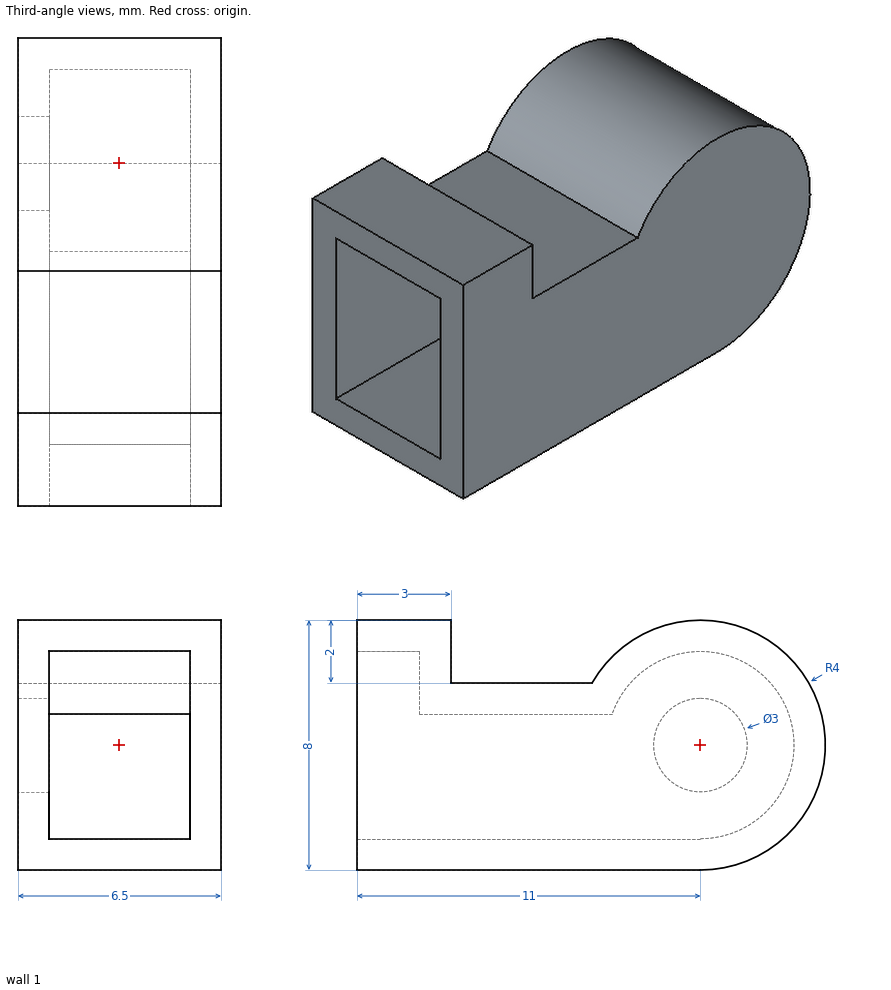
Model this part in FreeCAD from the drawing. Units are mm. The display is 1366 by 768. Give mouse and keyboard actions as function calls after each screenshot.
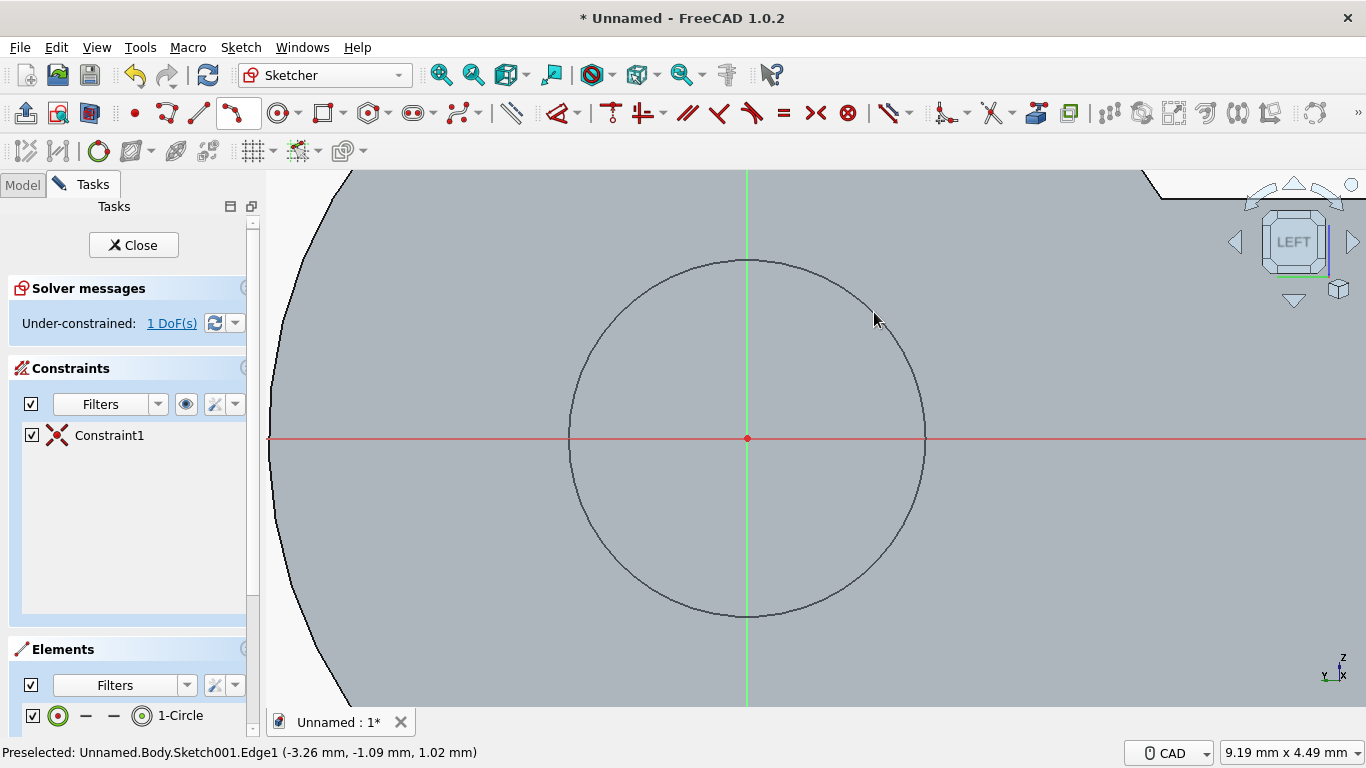
click(873, 312)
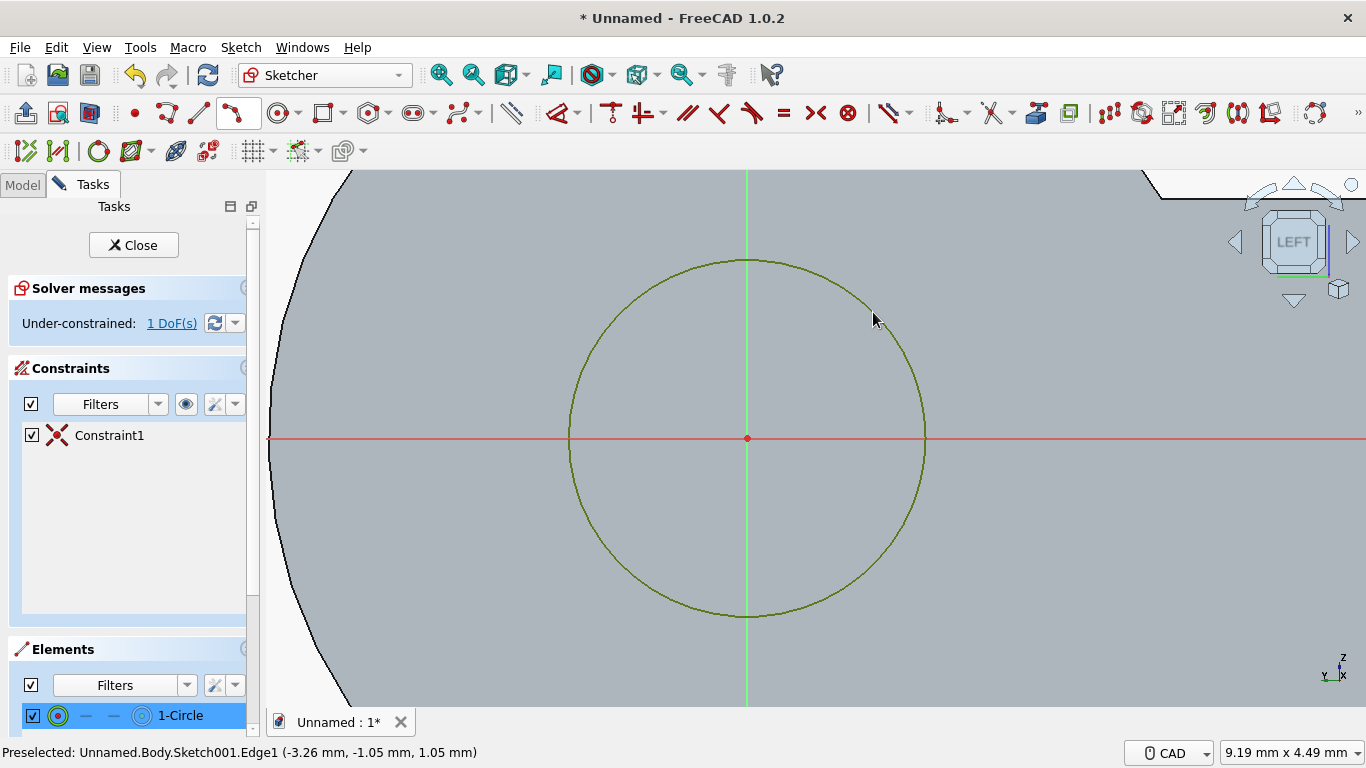
key(k)
key(o)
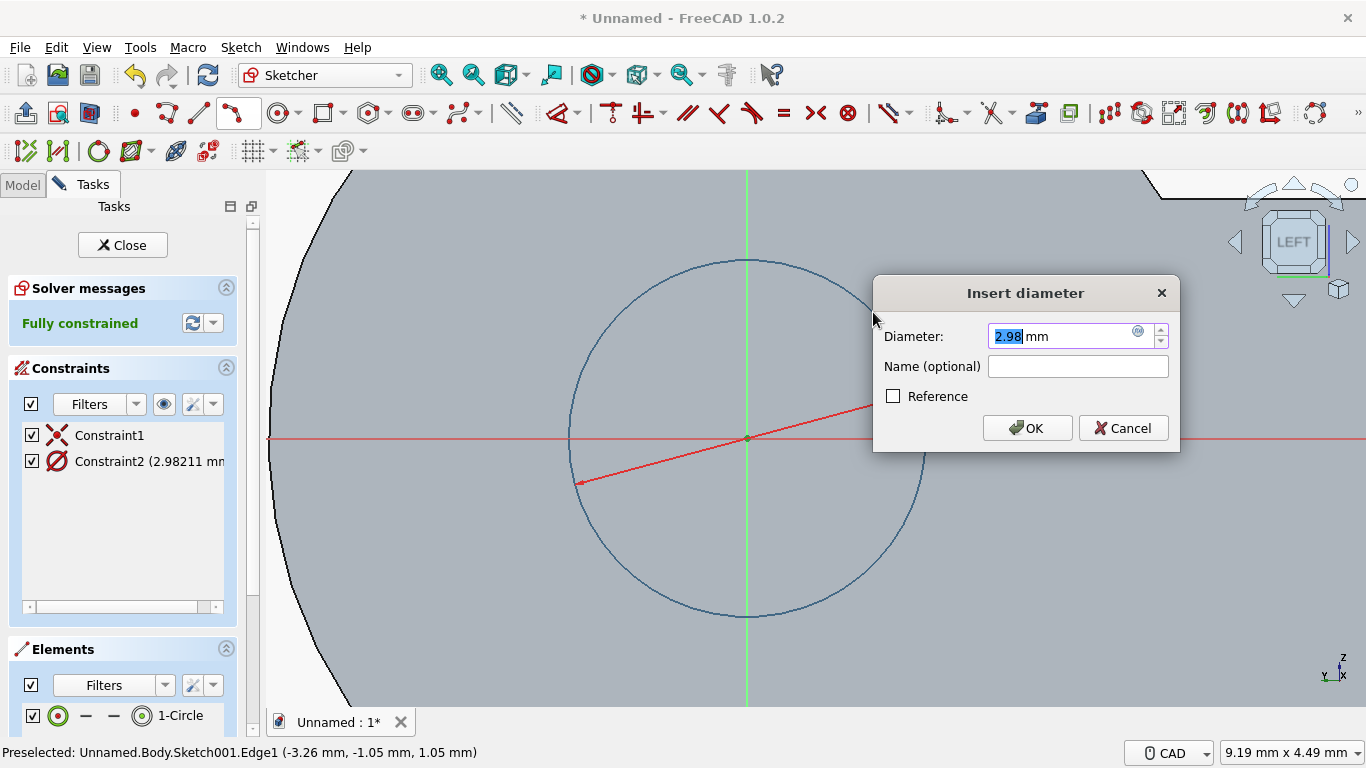
text(3)
key(Return)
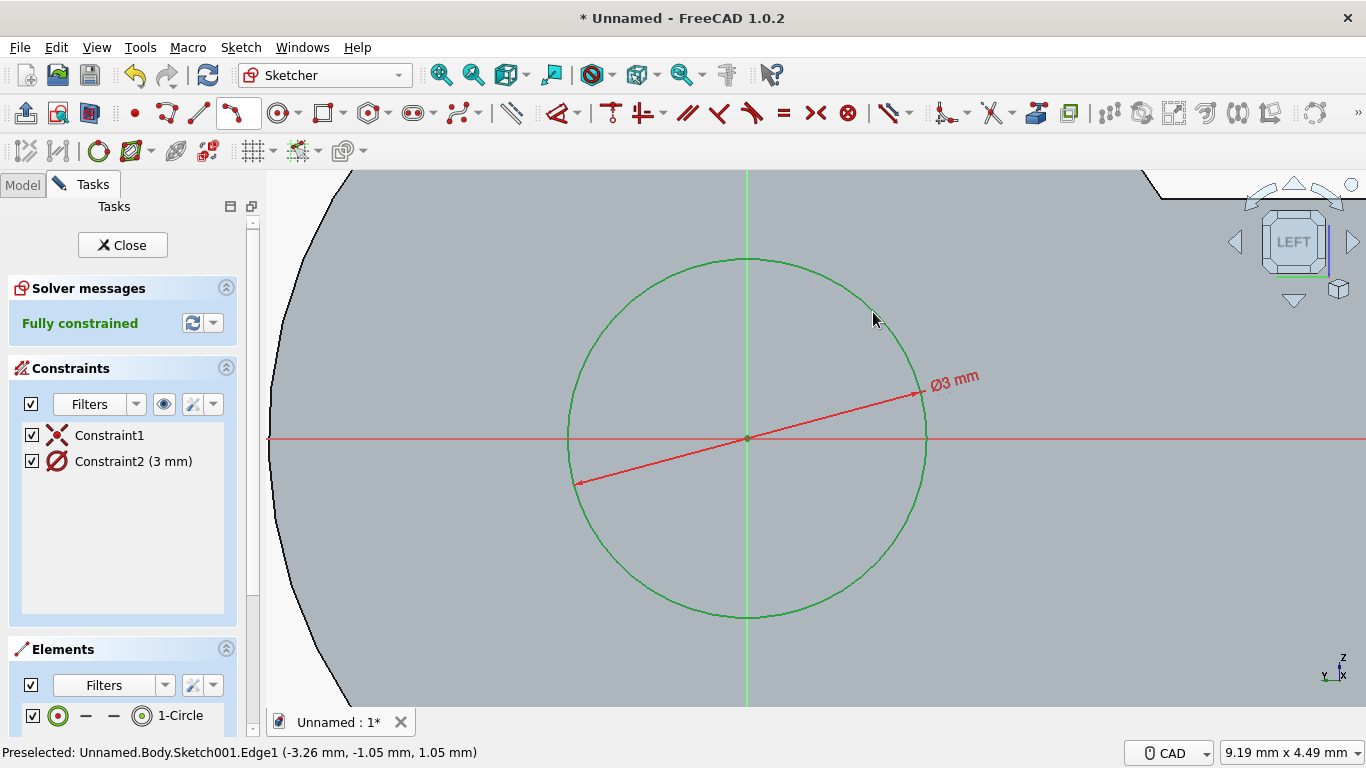
click(123, 245)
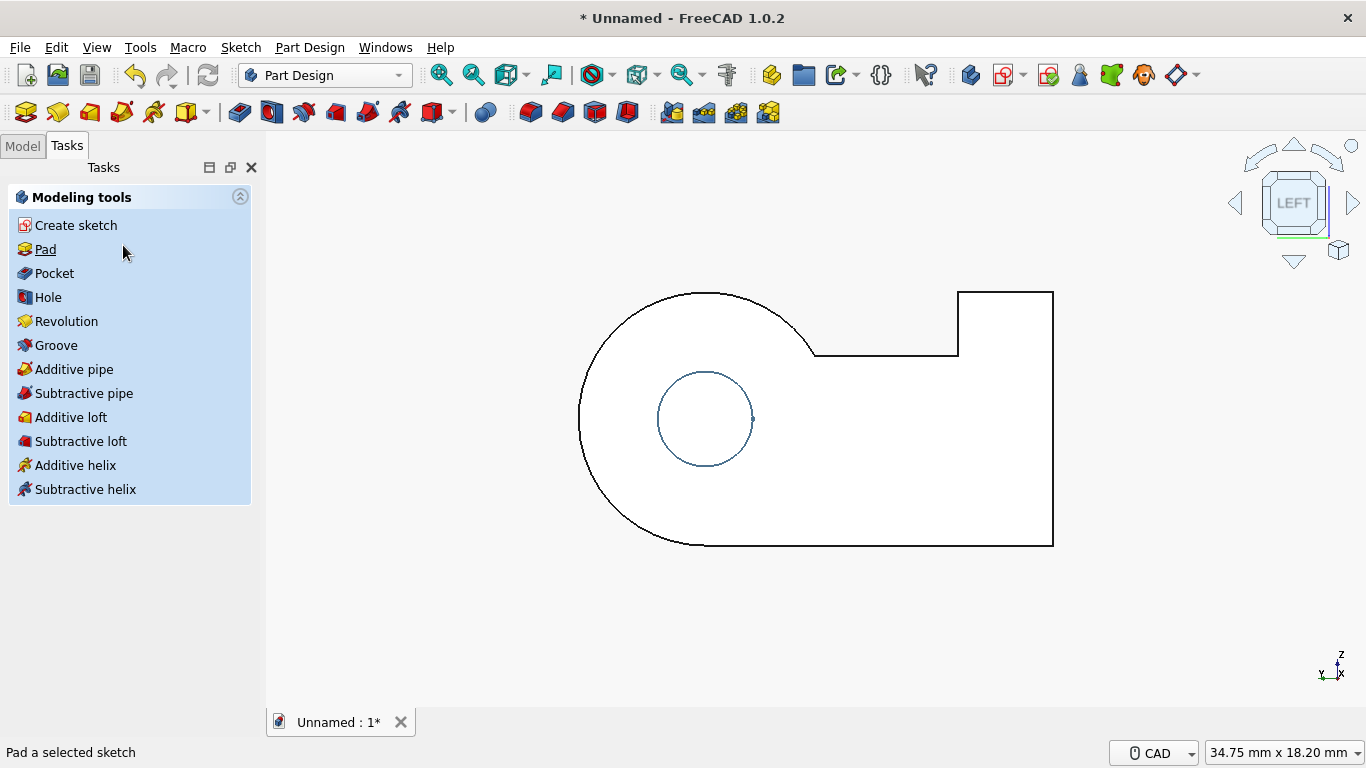
click(240, 112)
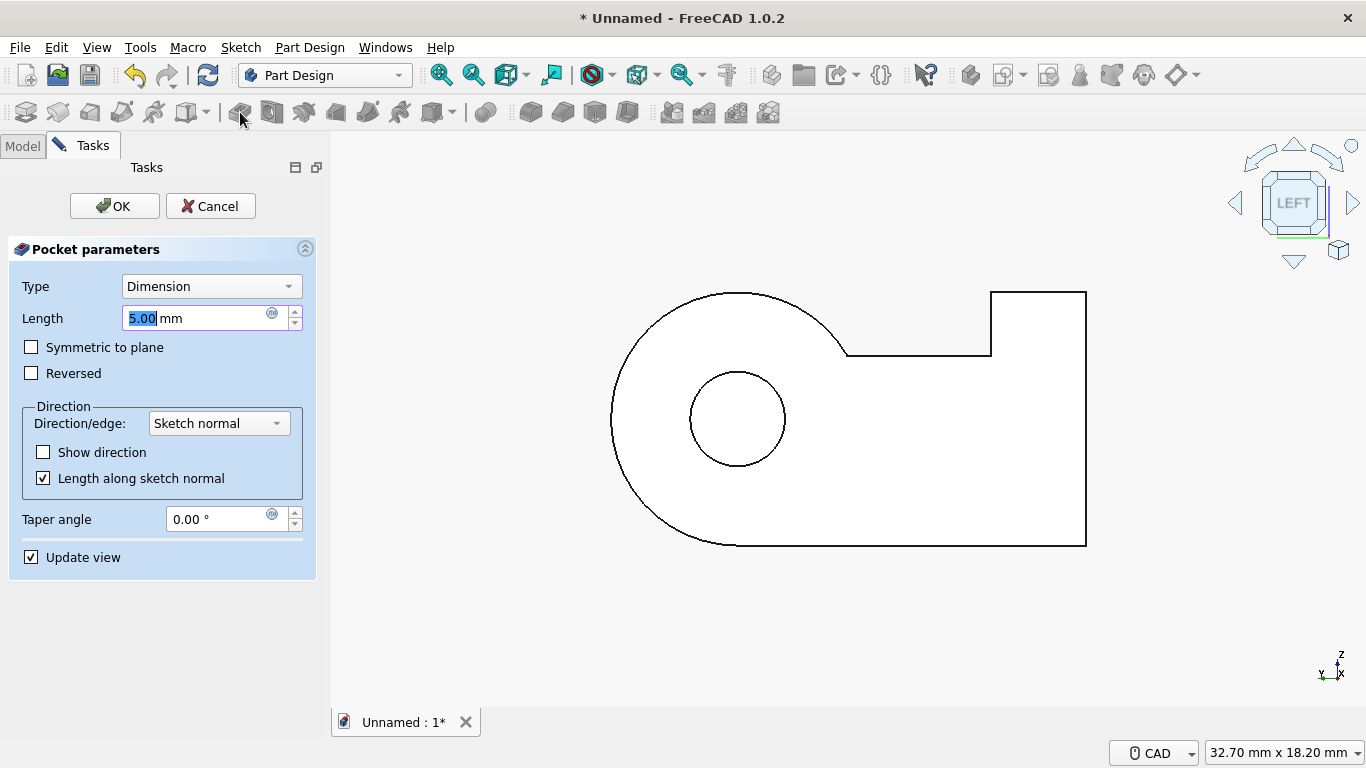
click(212, 286)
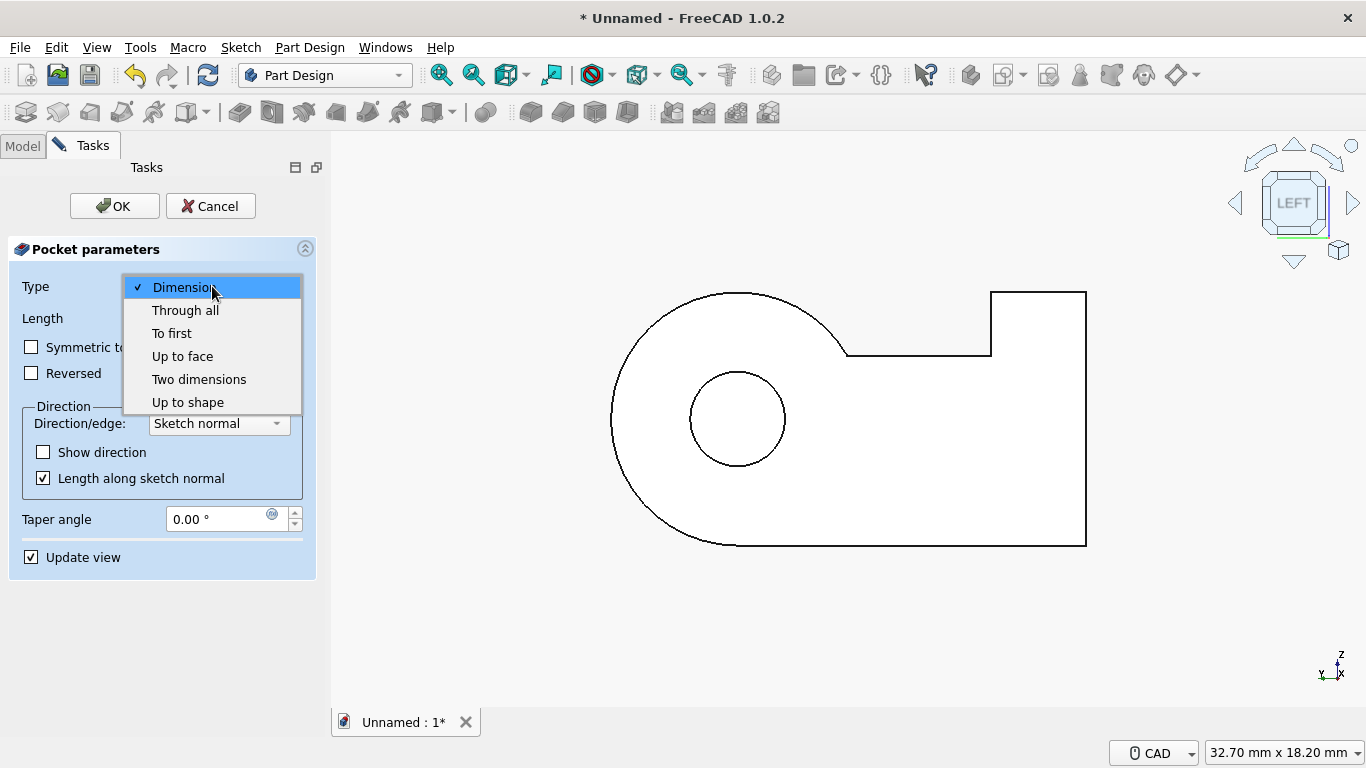
click(212, 334)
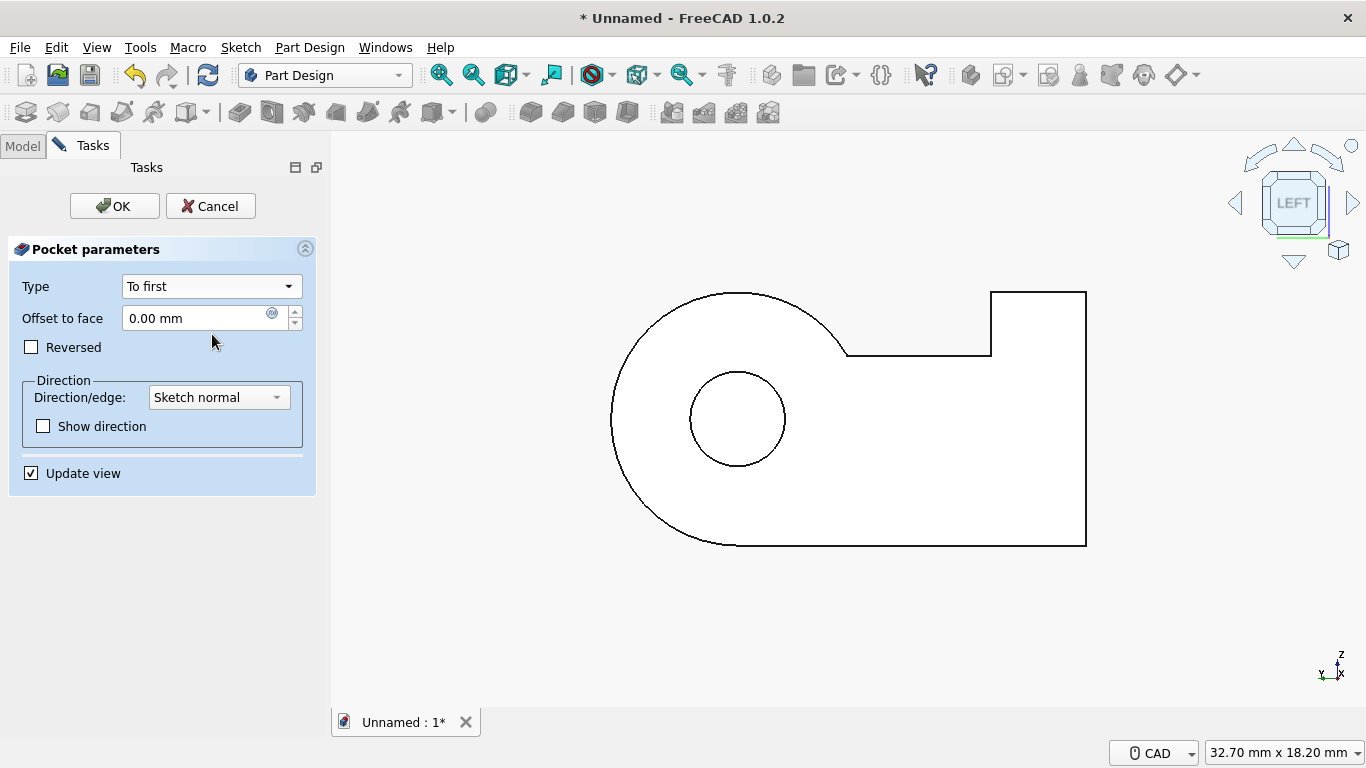
click(115, 206)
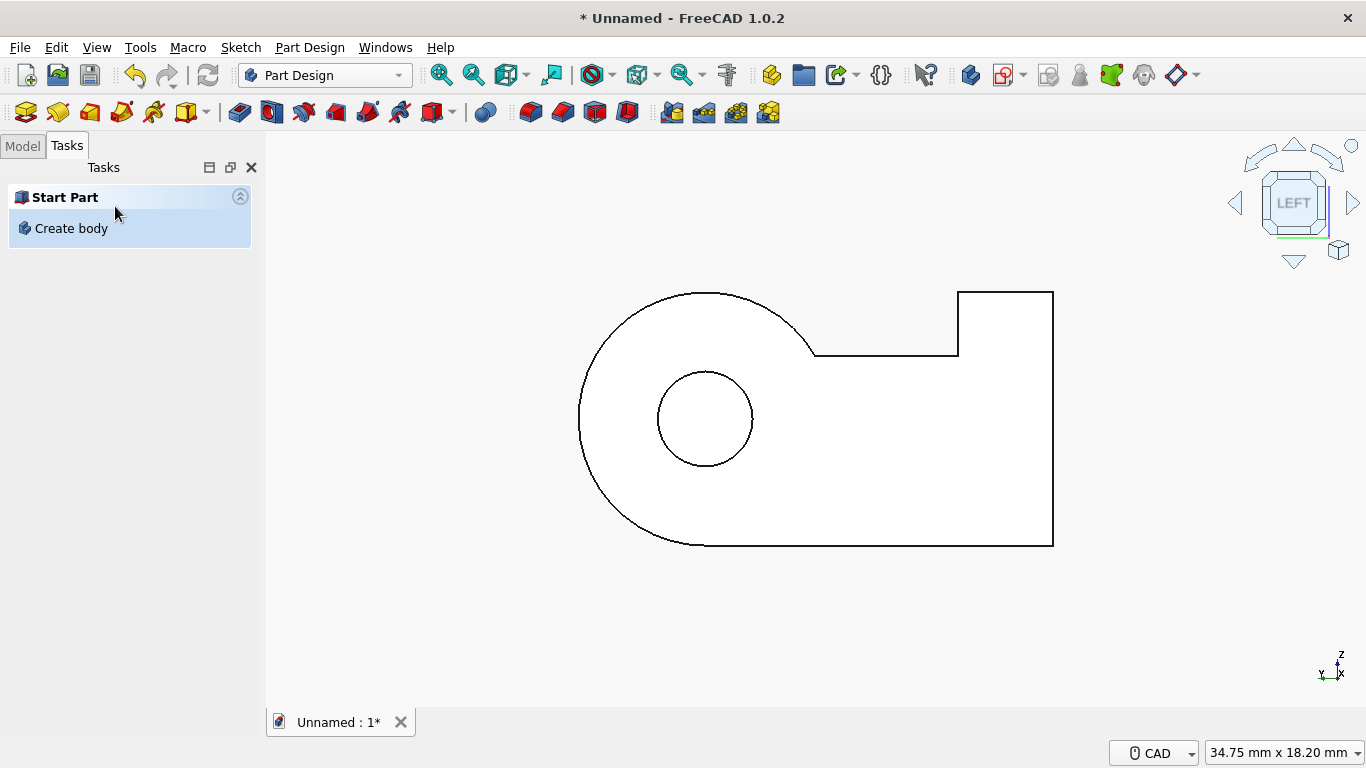
key(0)